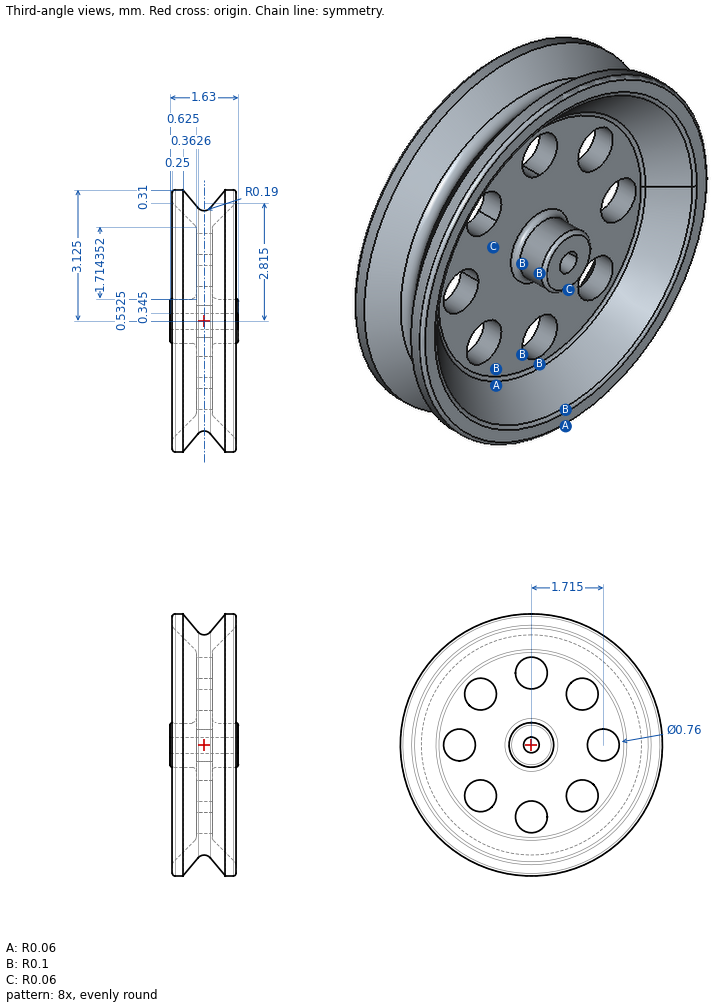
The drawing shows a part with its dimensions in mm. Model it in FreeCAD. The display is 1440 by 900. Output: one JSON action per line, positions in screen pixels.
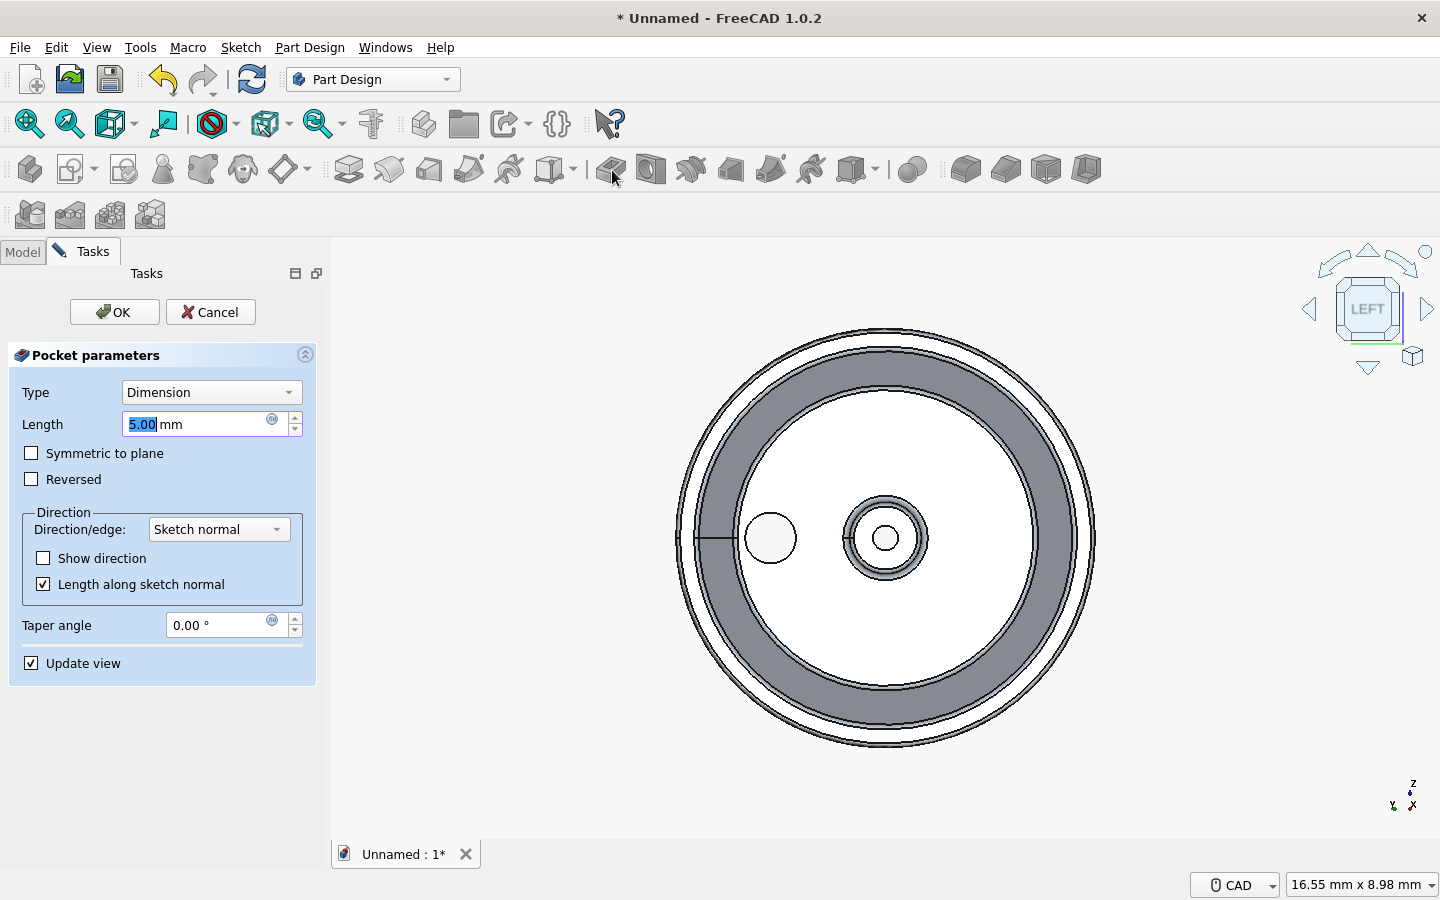
{"action": "left_click", "coordinate": [212, 392]}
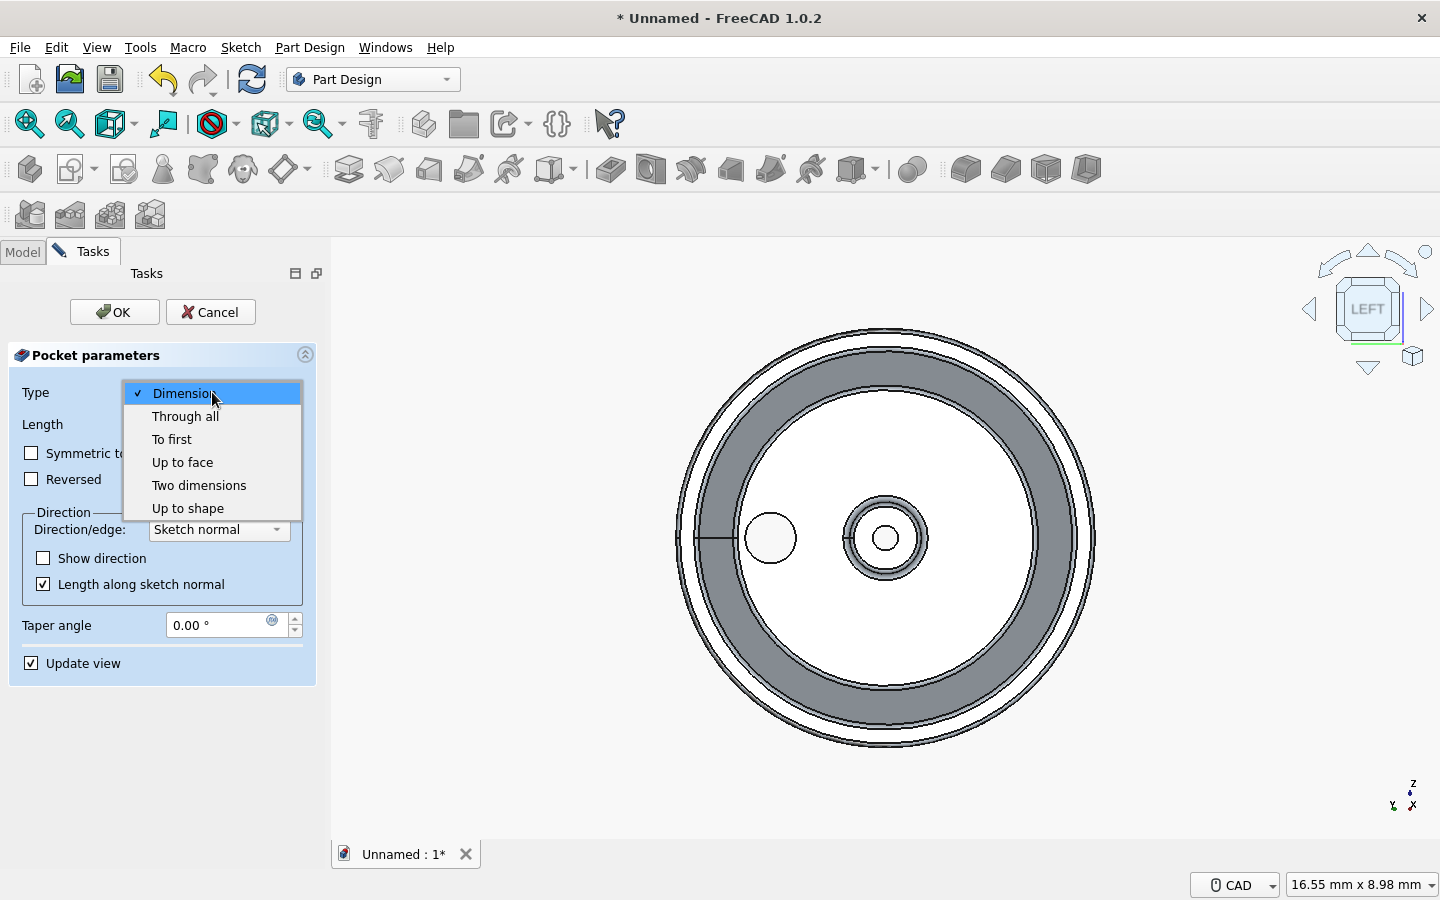
{"action": "left_click", "coordinate": [212, 416]}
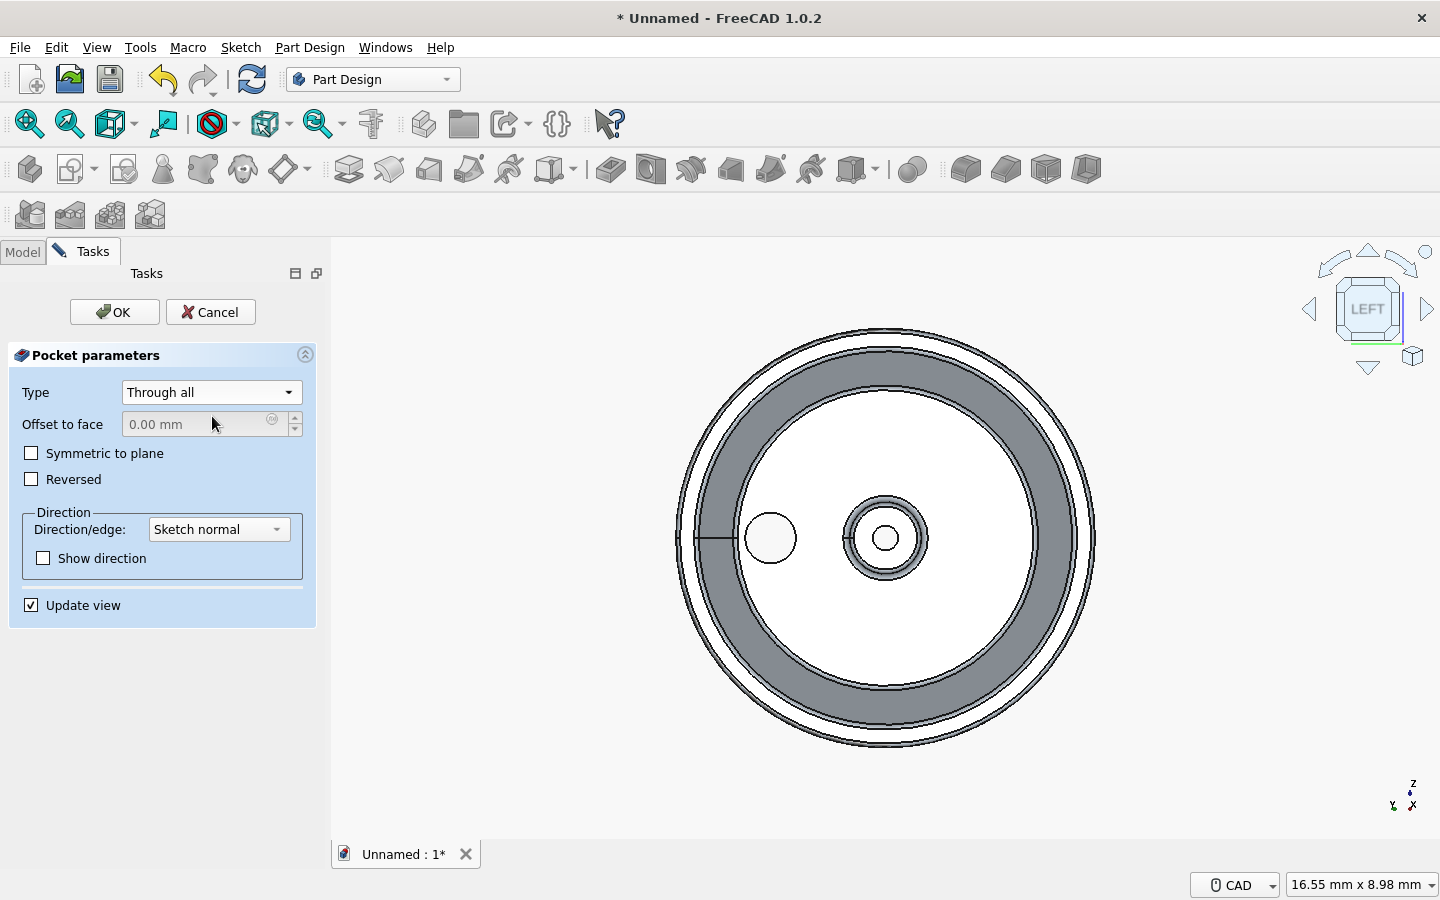
{"action": "left_click", "coordinate": [115, 312]}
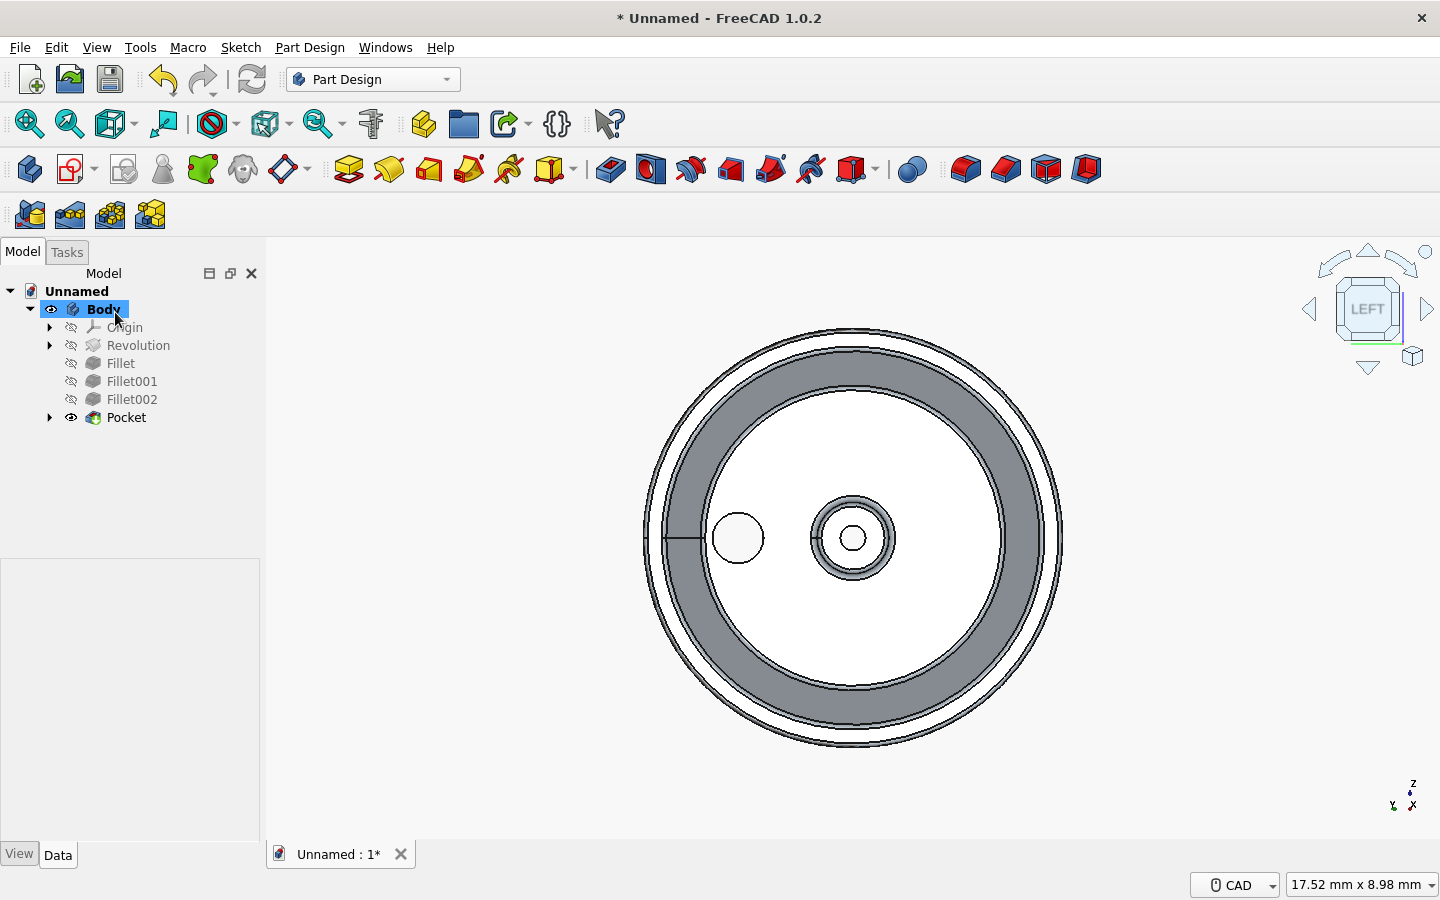
{"action": "left_click", "coordinate": [116, 417]}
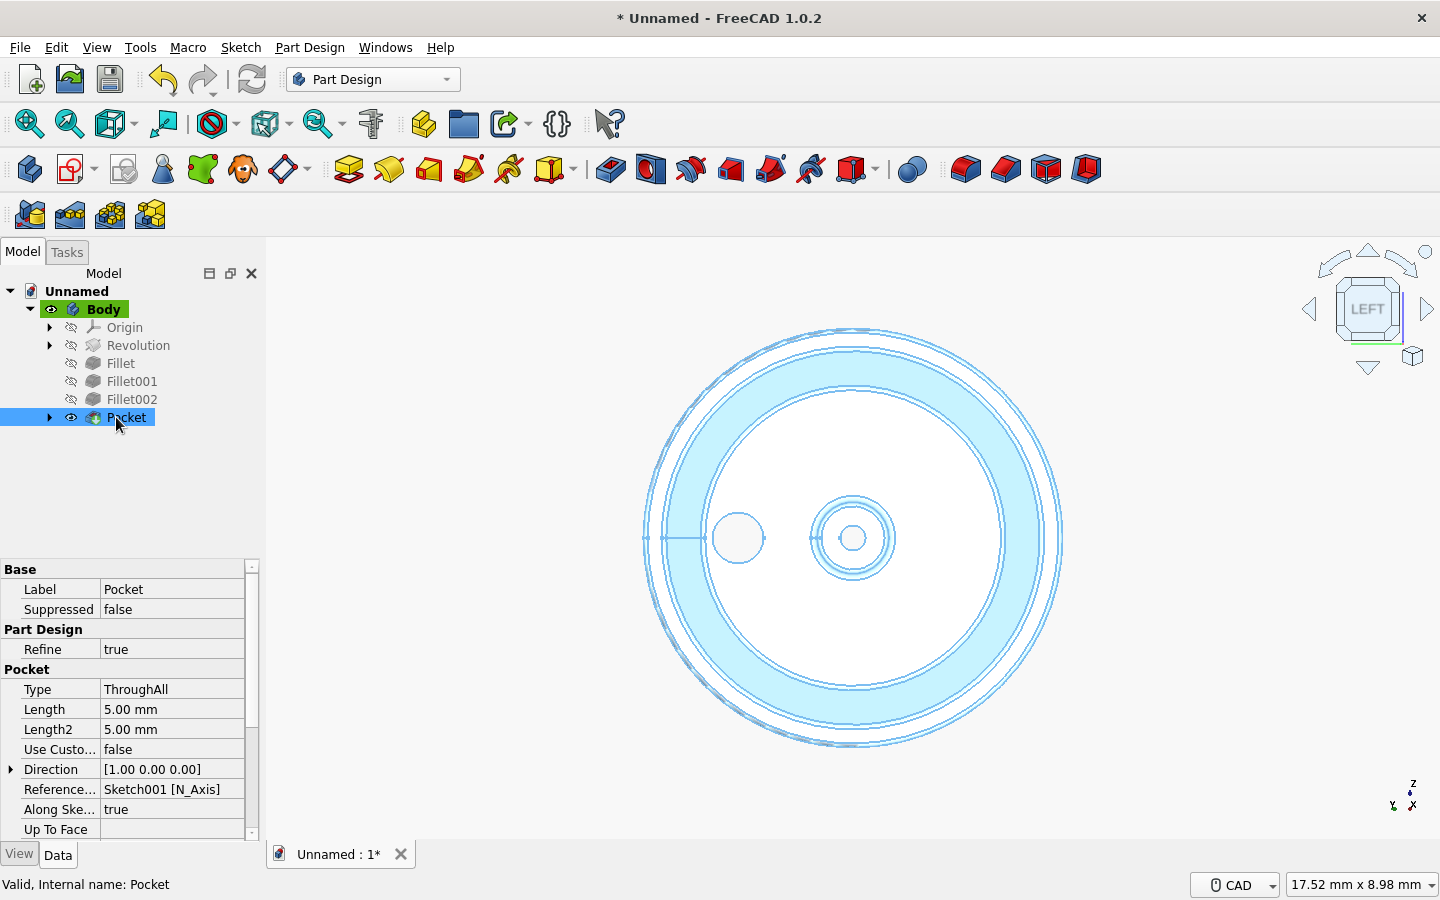
{"action": "left_click", "coordinate": [110, 214]}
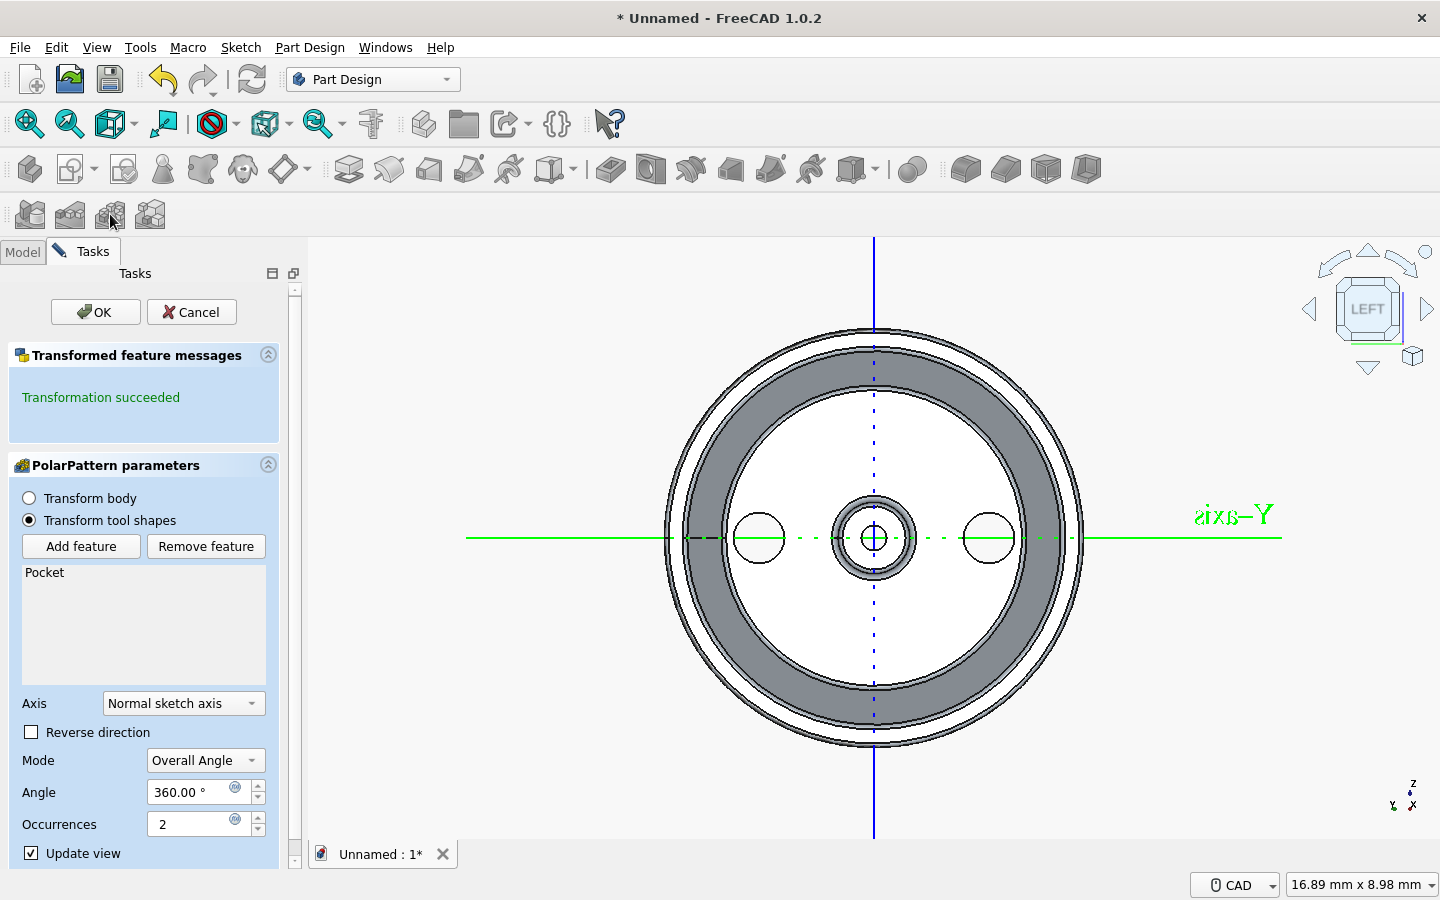
{"action": "left_click", "coordinate": [184, 704]}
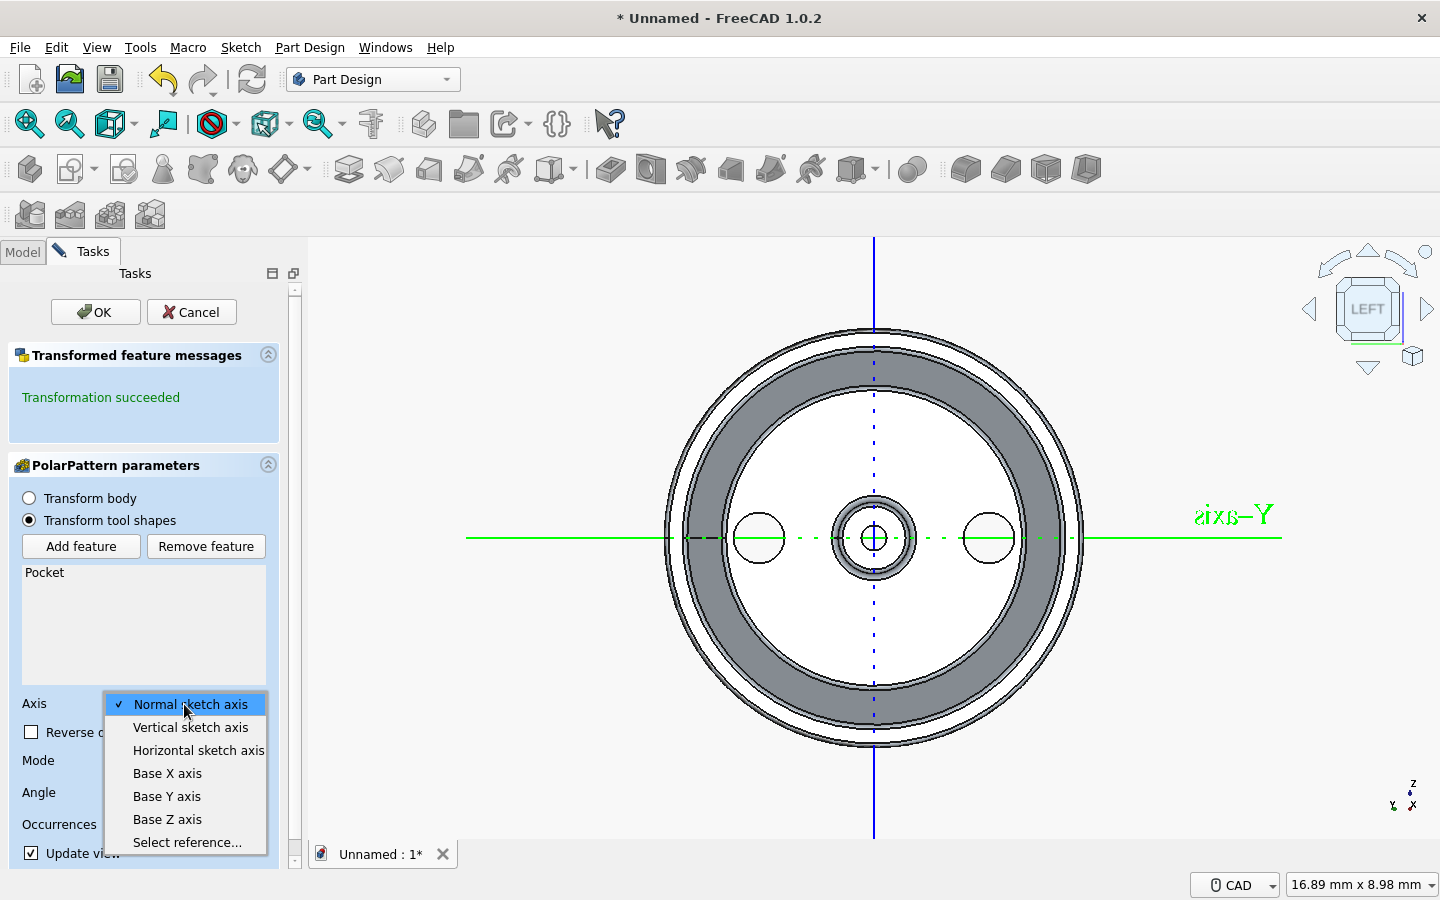
{"action": "left_click", "coordinate": [184, 774]}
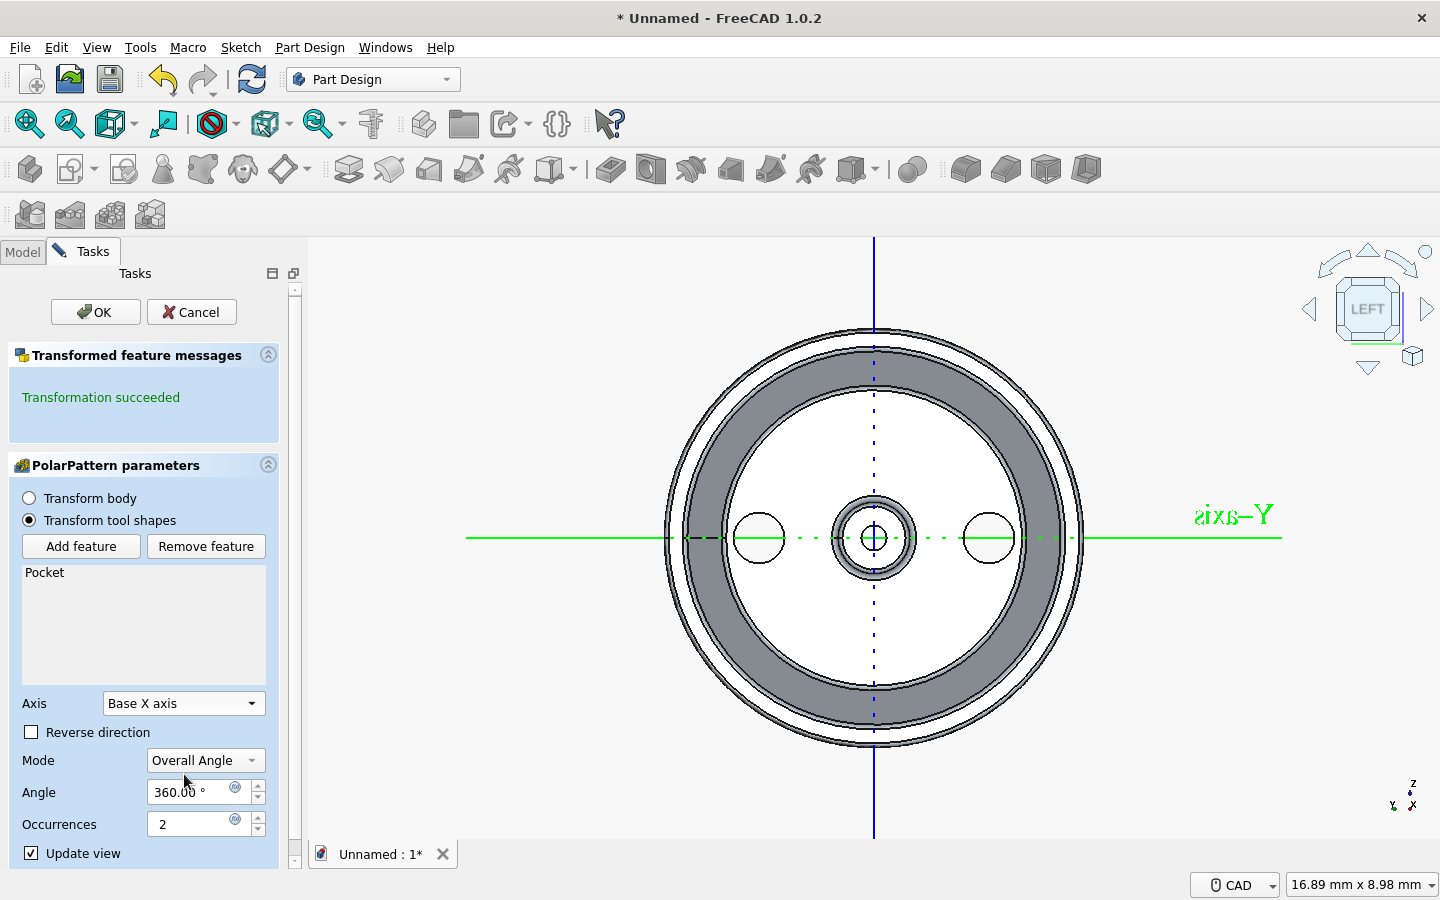
{"action": "triple_click", "coordinate": [198, 824]}